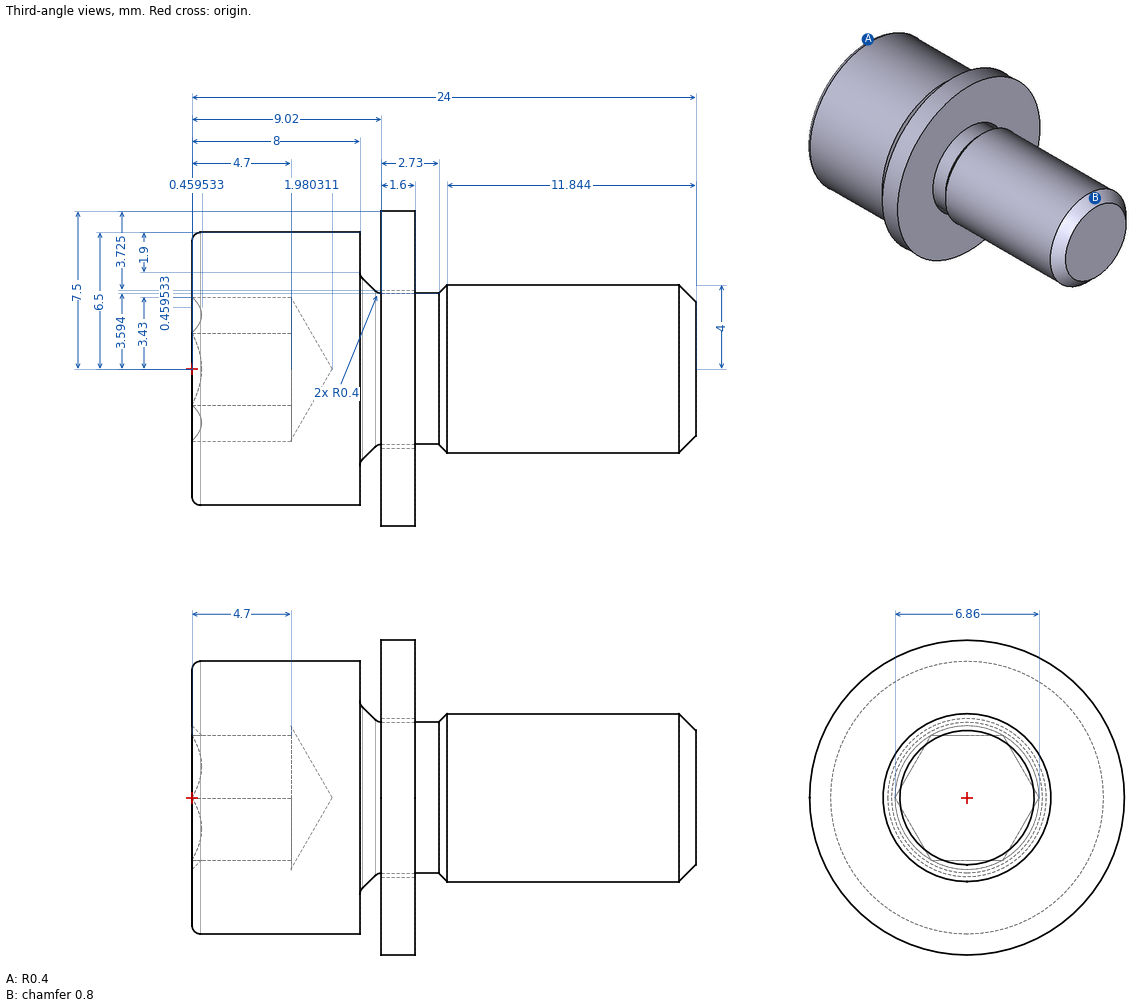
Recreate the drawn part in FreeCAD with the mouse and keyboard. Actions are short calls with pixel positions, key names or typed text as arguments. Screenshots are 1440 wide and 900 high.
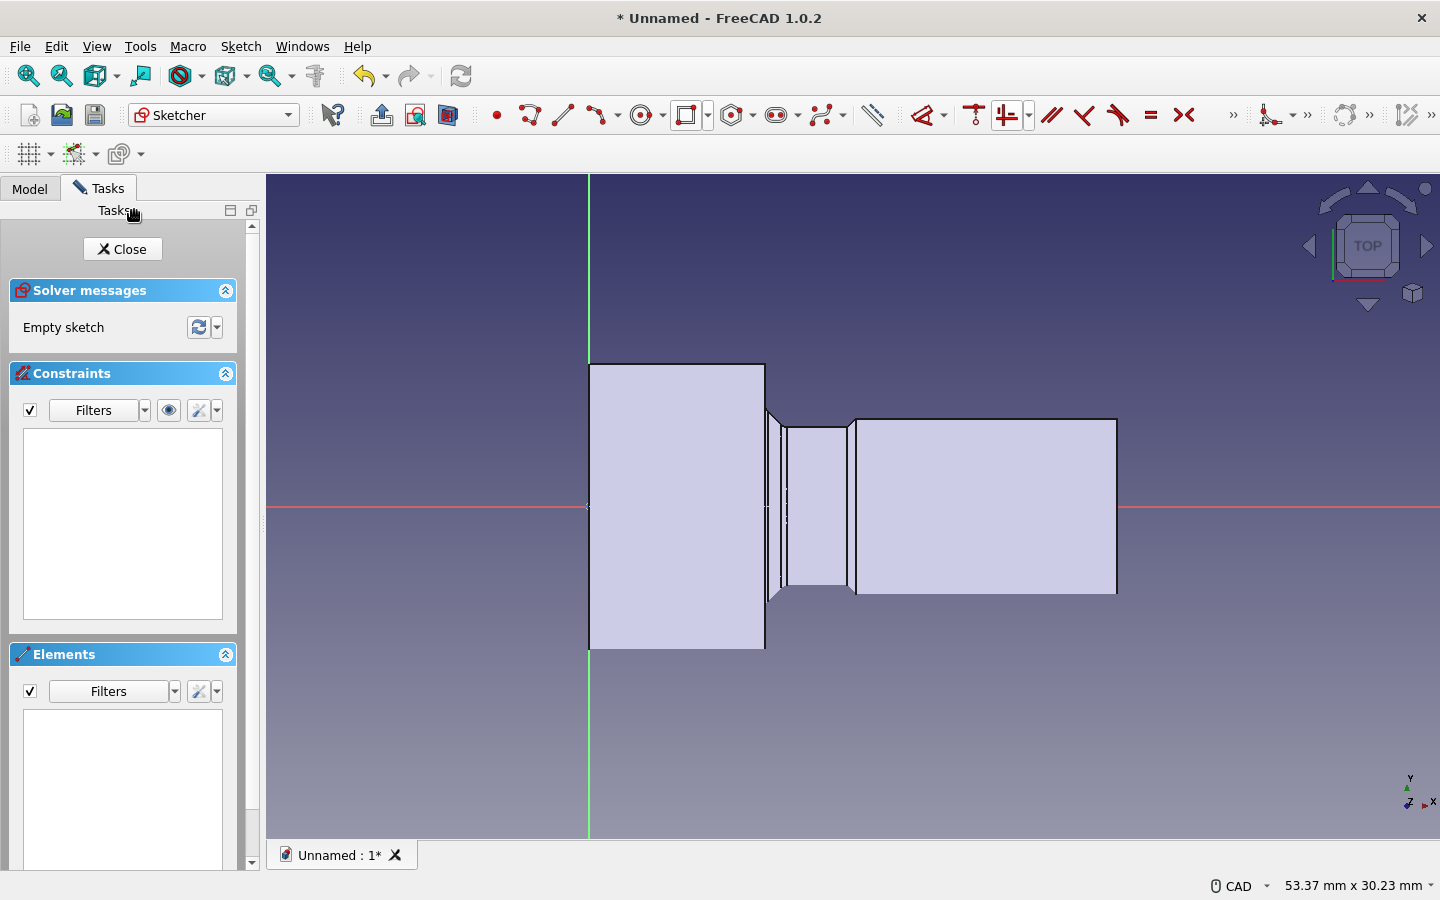
click(448, 116)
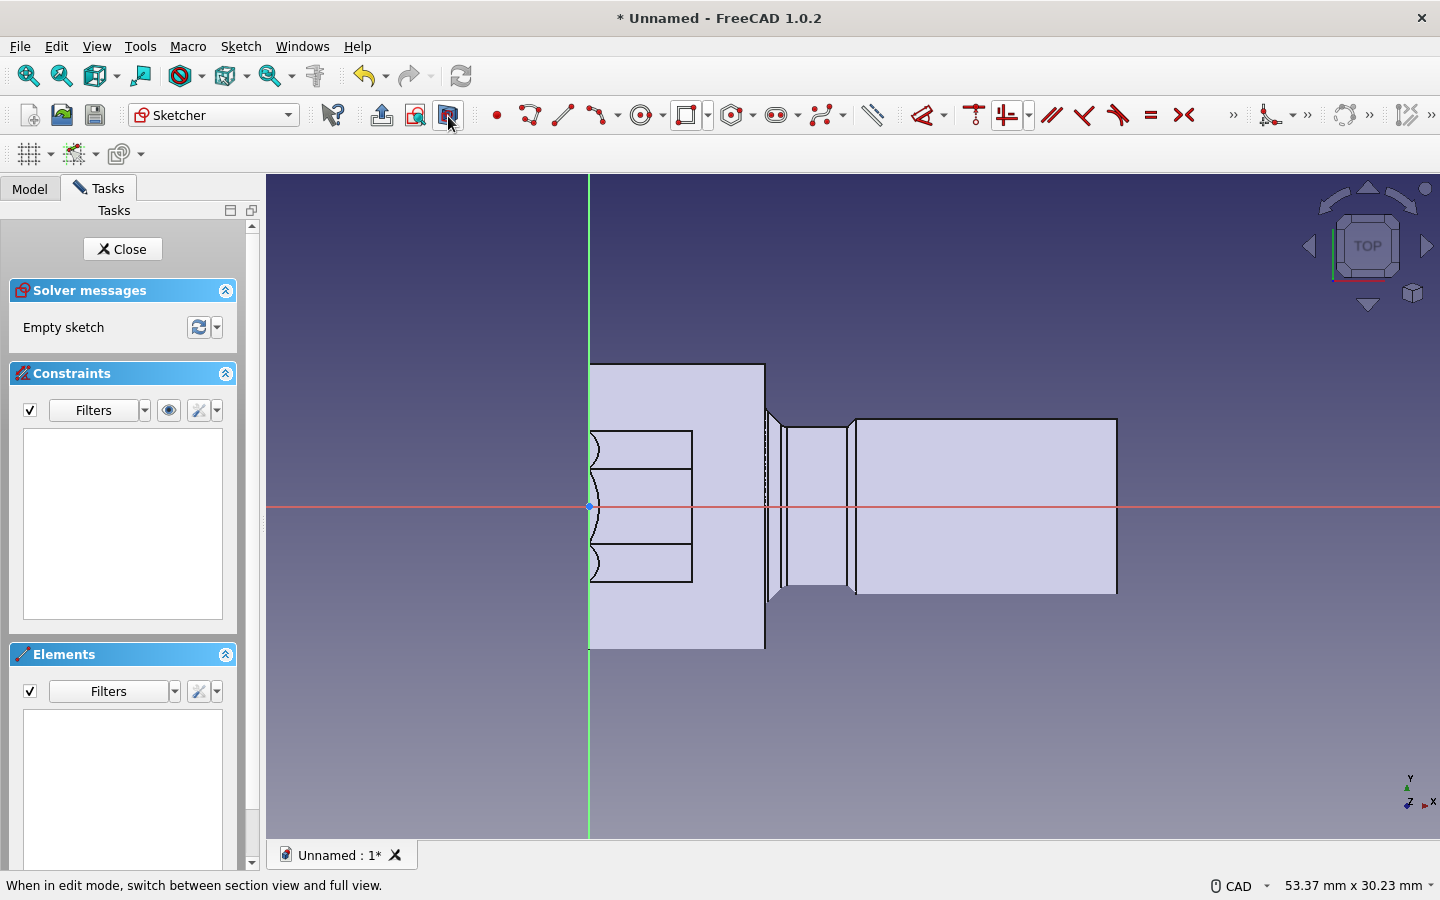
scroll(632, 459, up, 8)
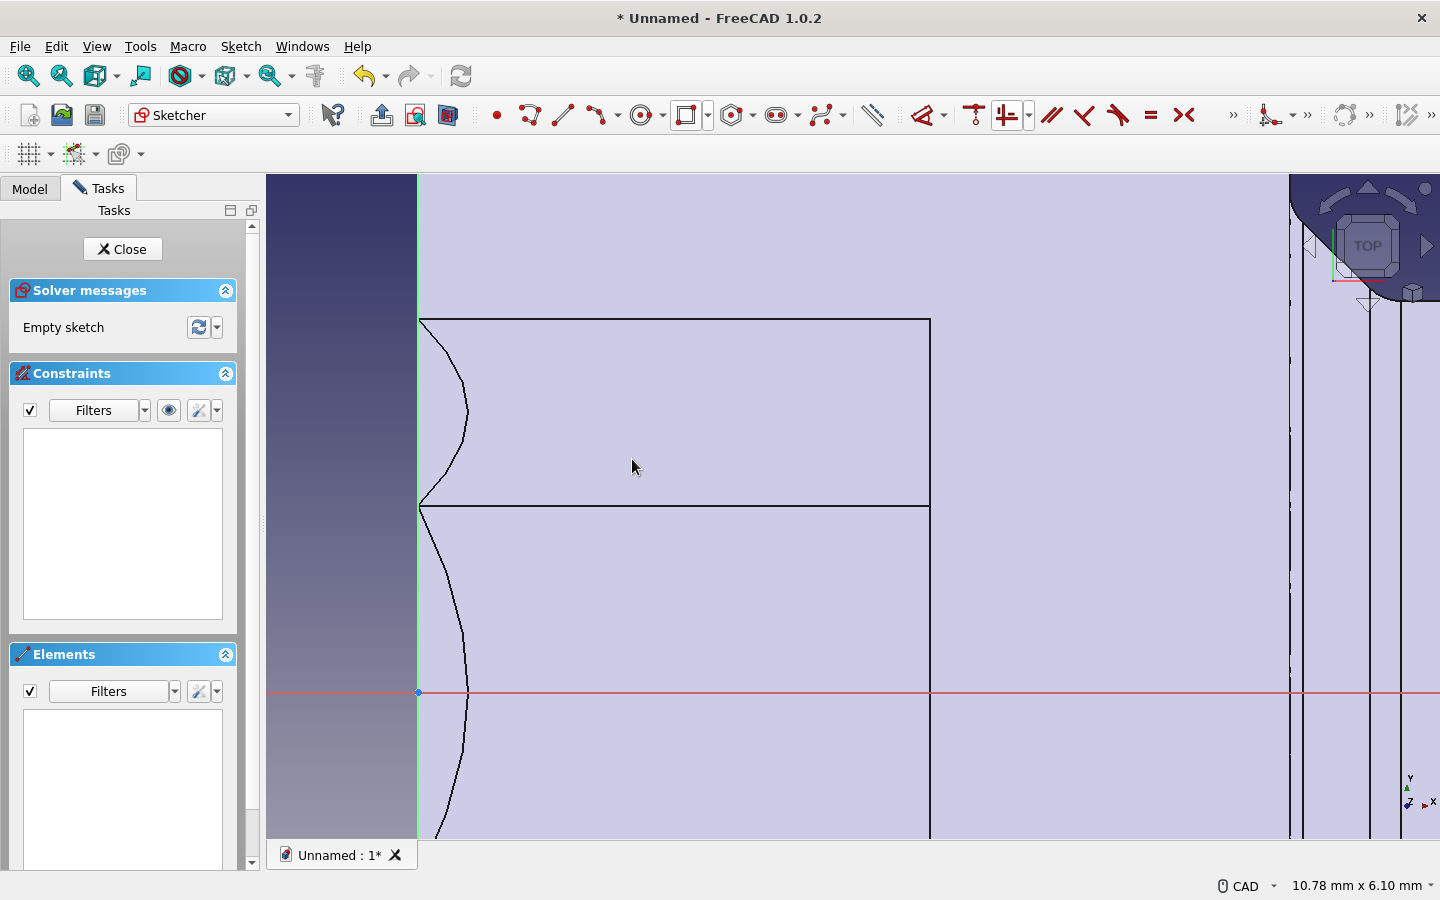
click(530, 116)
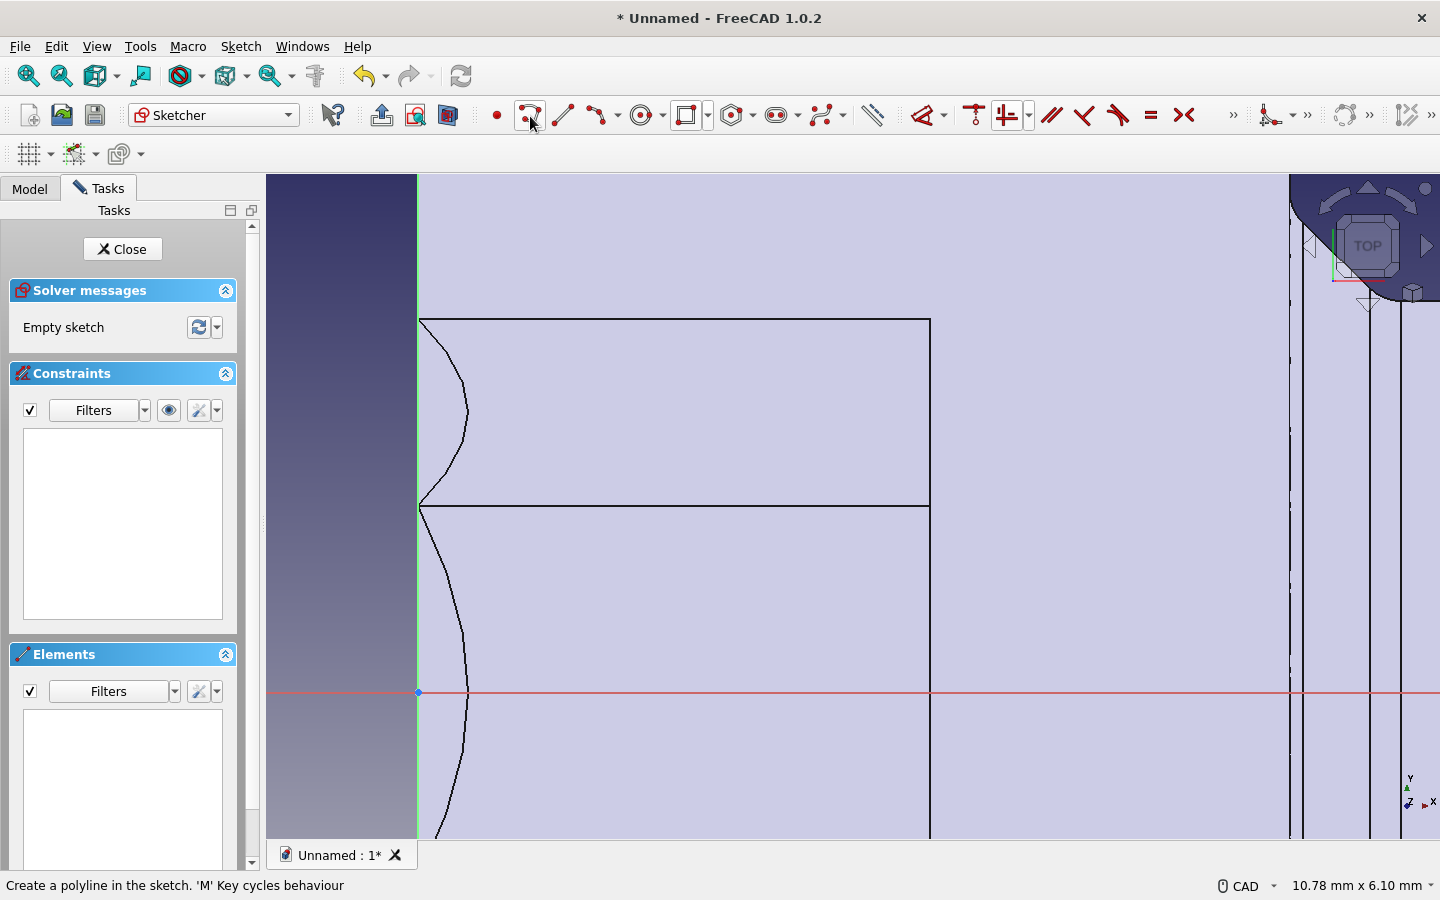
click(930, 693)
click(1146, 684)
click(930, 319)
click(930, 693)
key(Escape)
key(Escape)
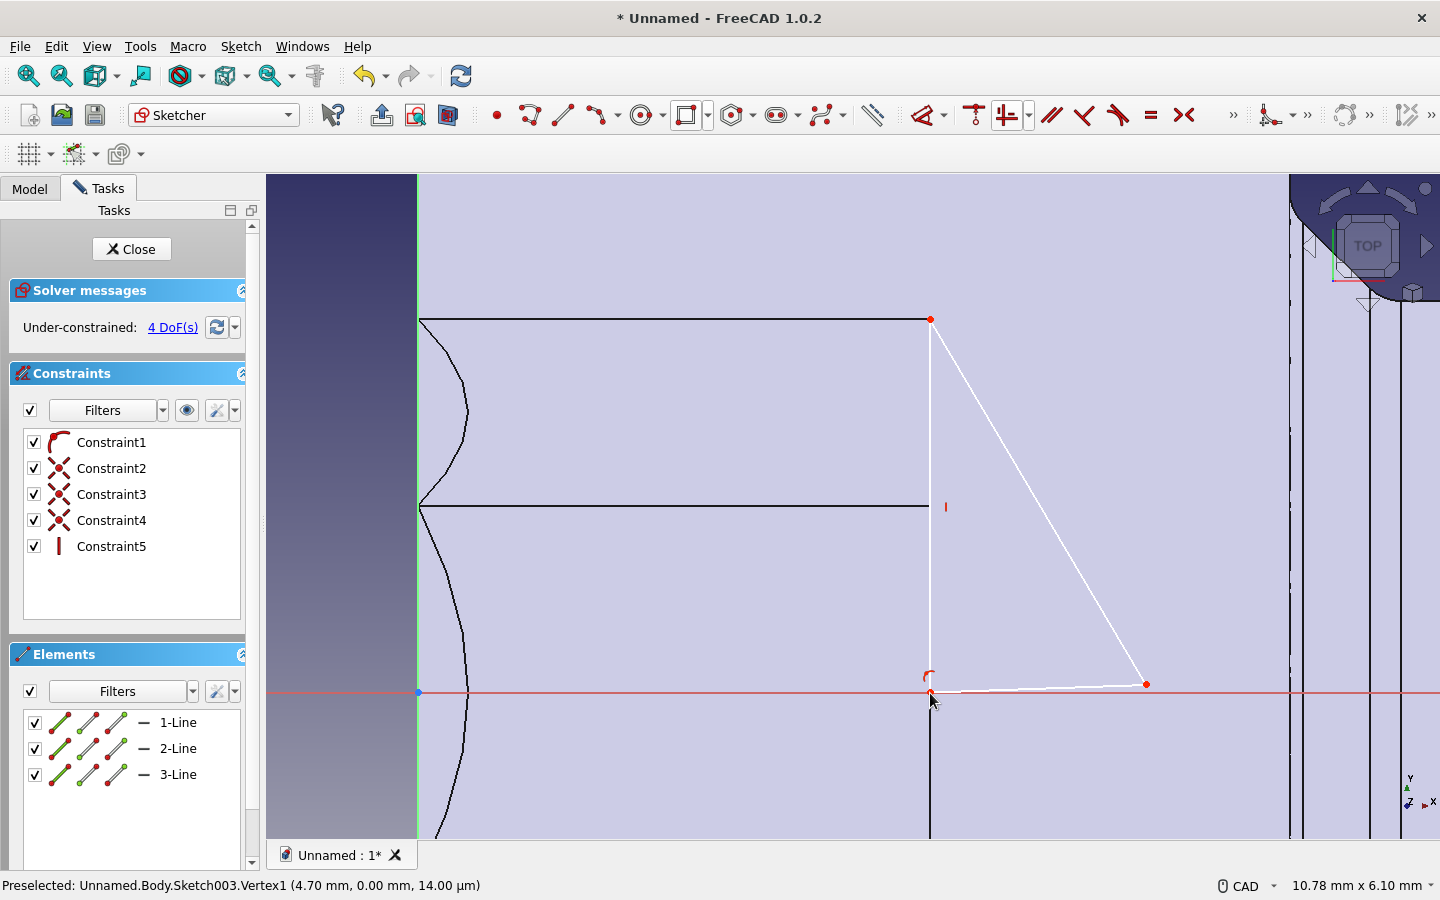
click(995, 690)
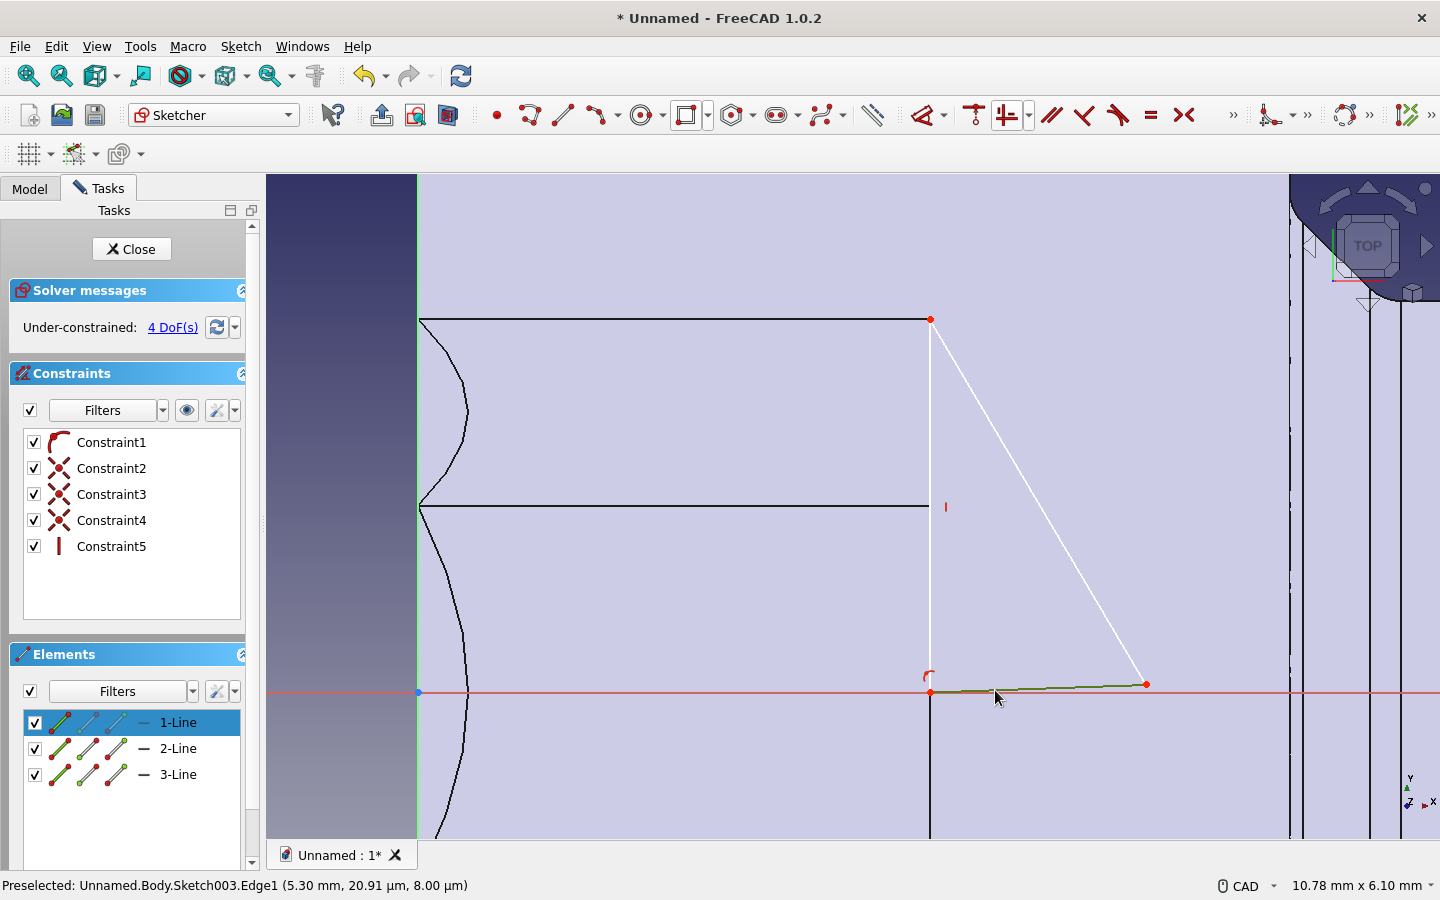
key(h)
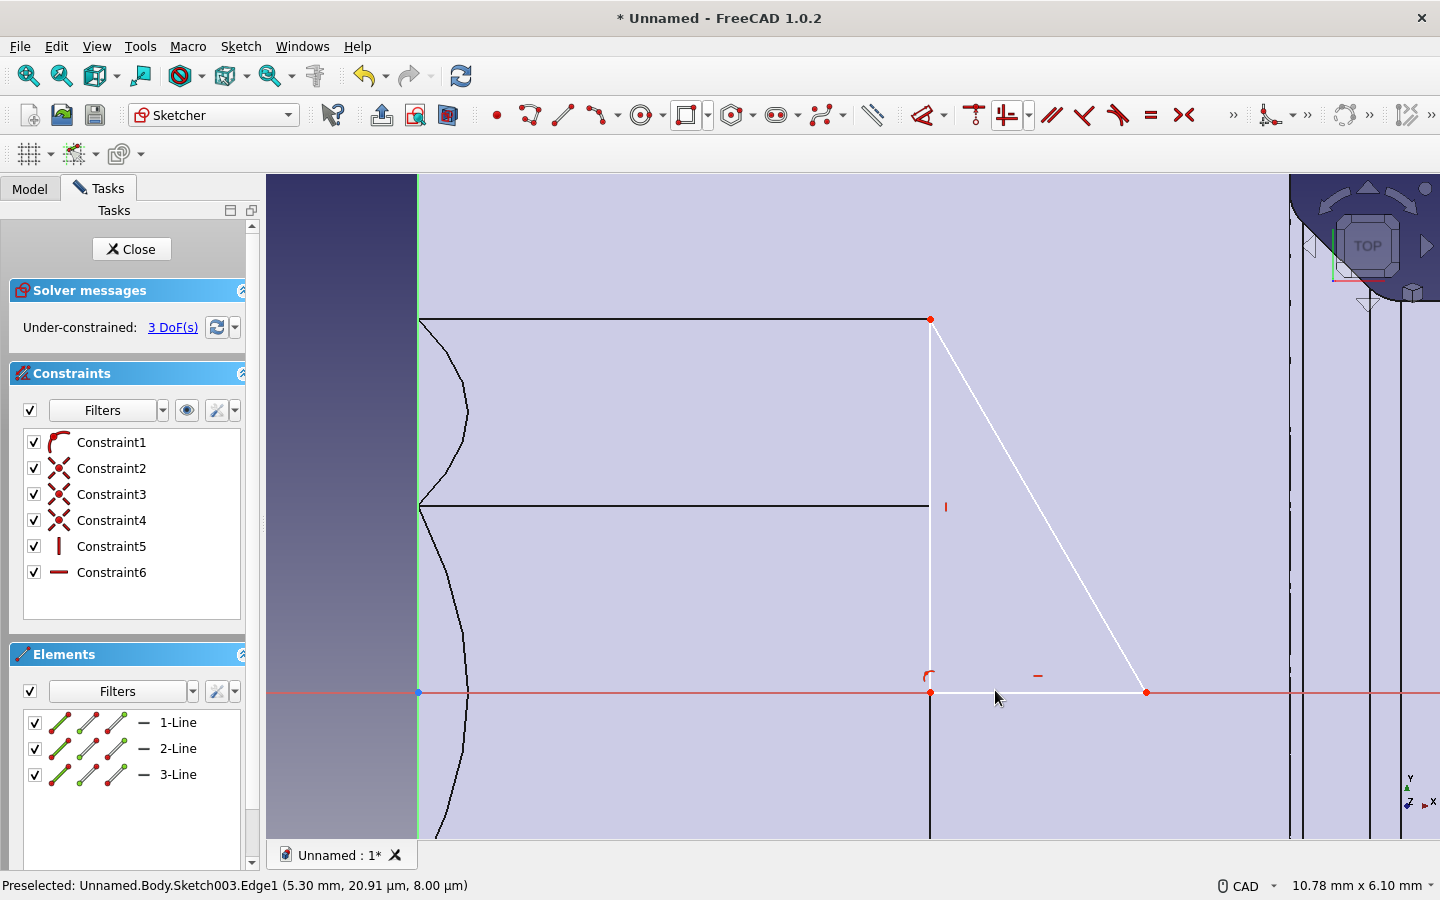
click(922, 116)